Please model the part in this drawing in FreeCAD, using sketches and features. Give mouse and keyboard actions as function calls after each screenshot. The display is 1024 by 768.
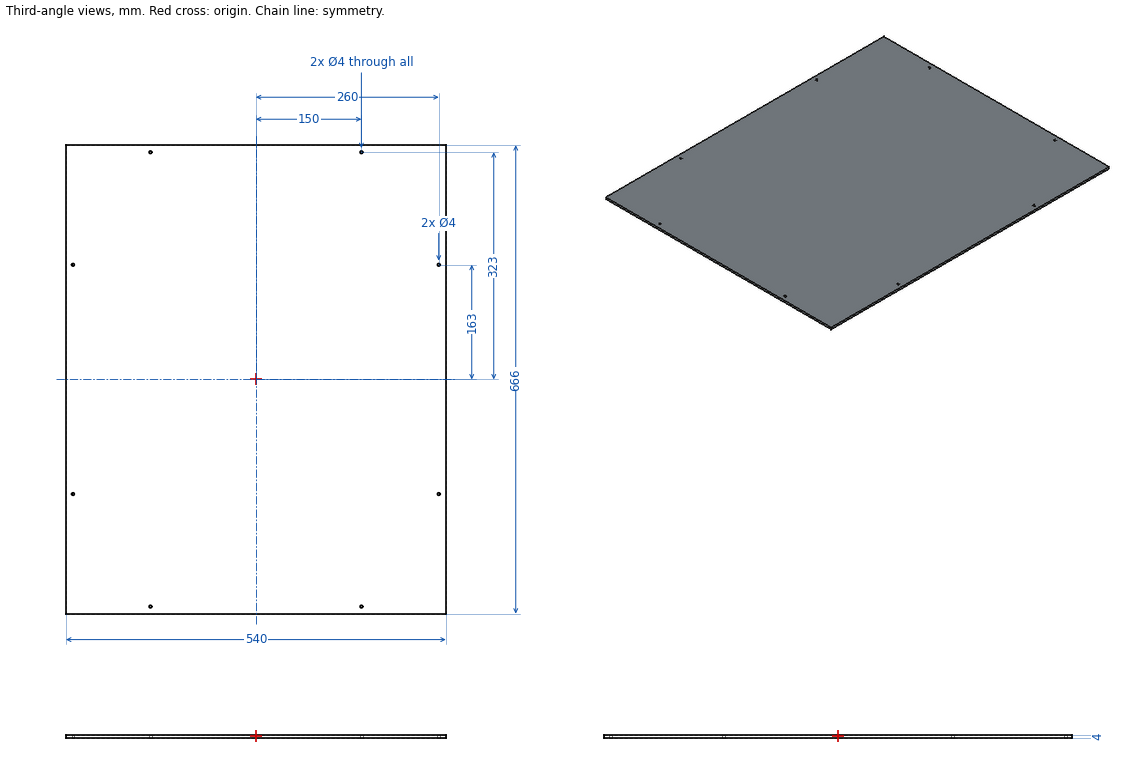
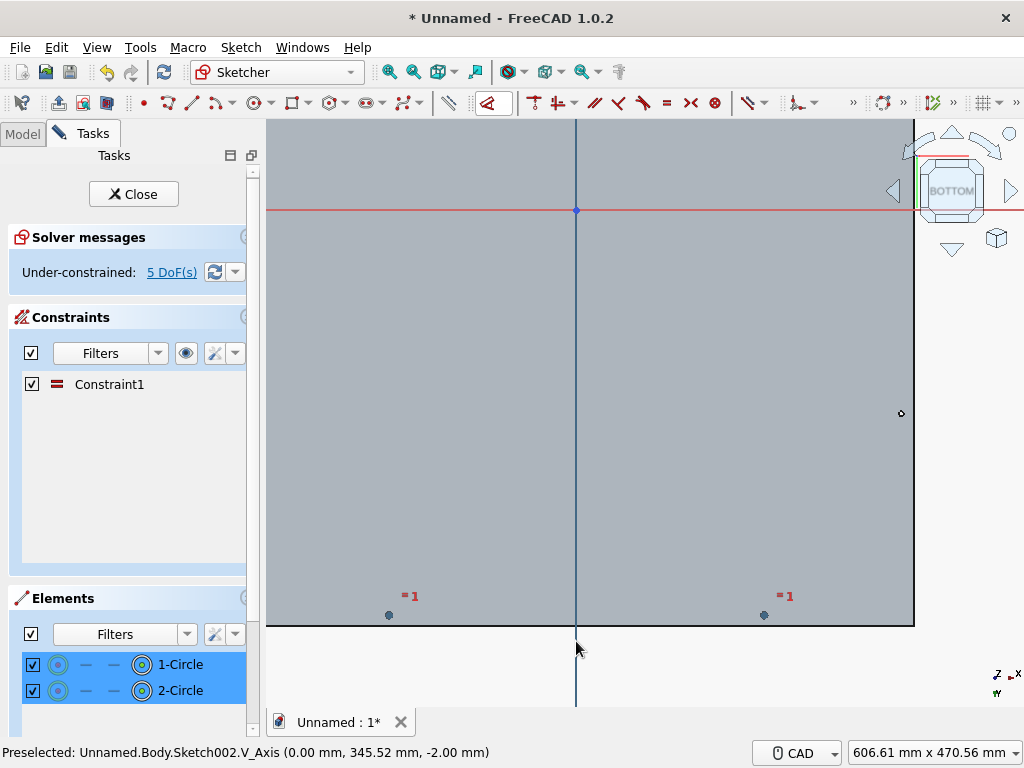
key(s)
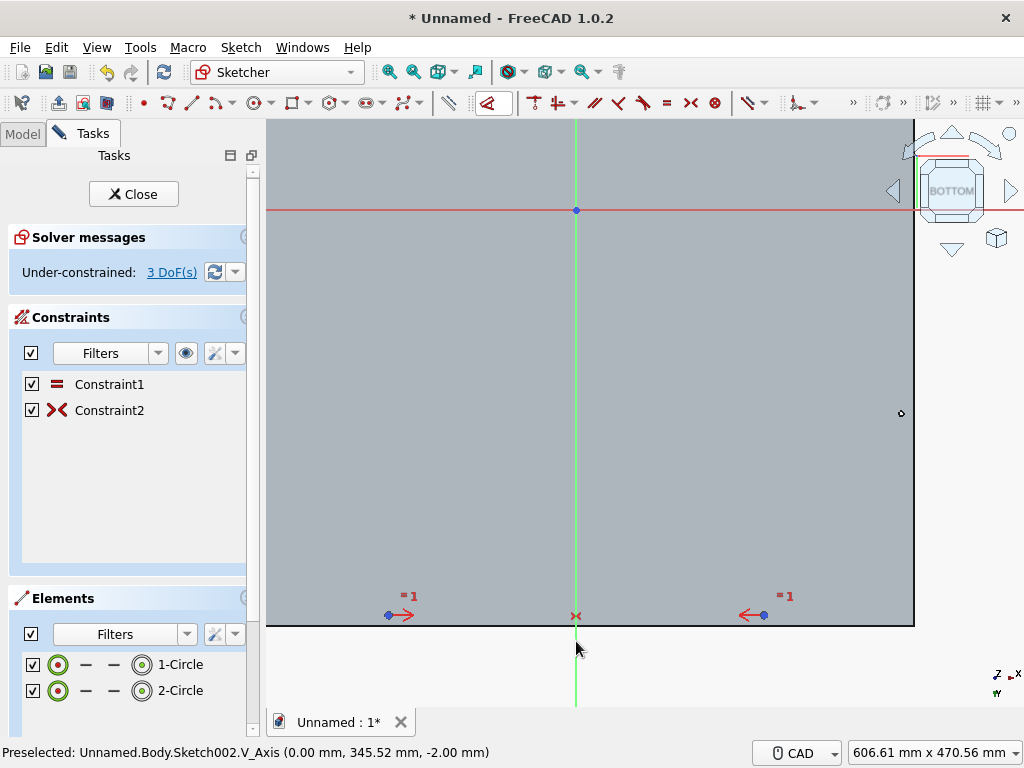
scroll(766, 613, up, 11)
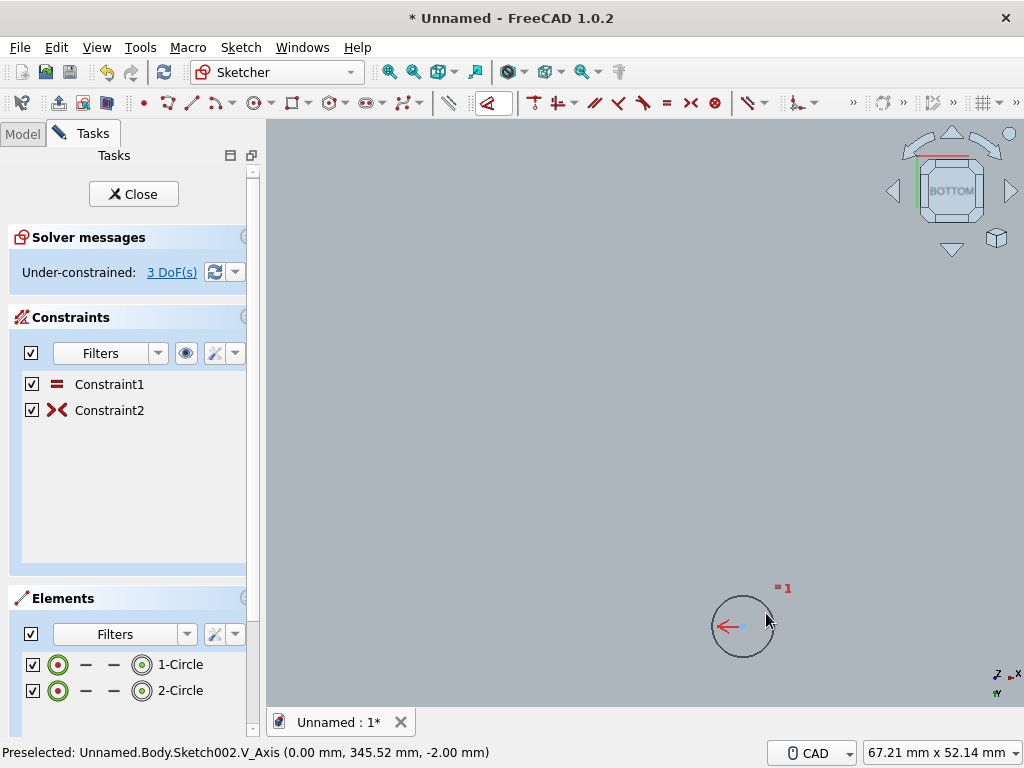
click(765, 605)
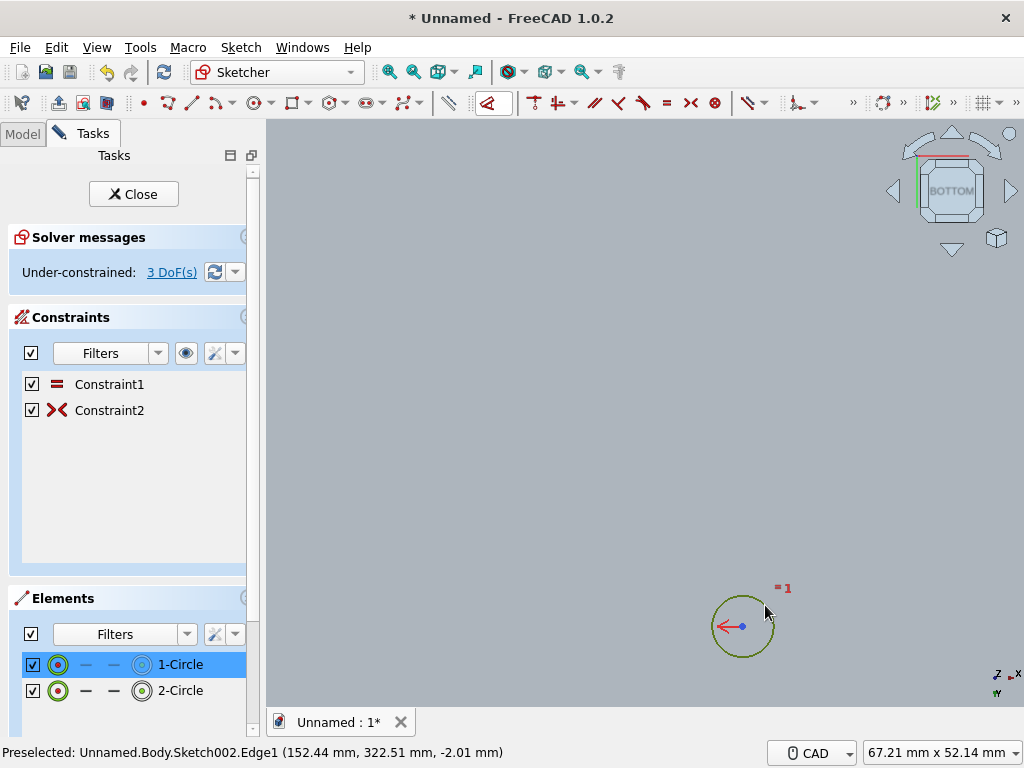
key(k)
key(o)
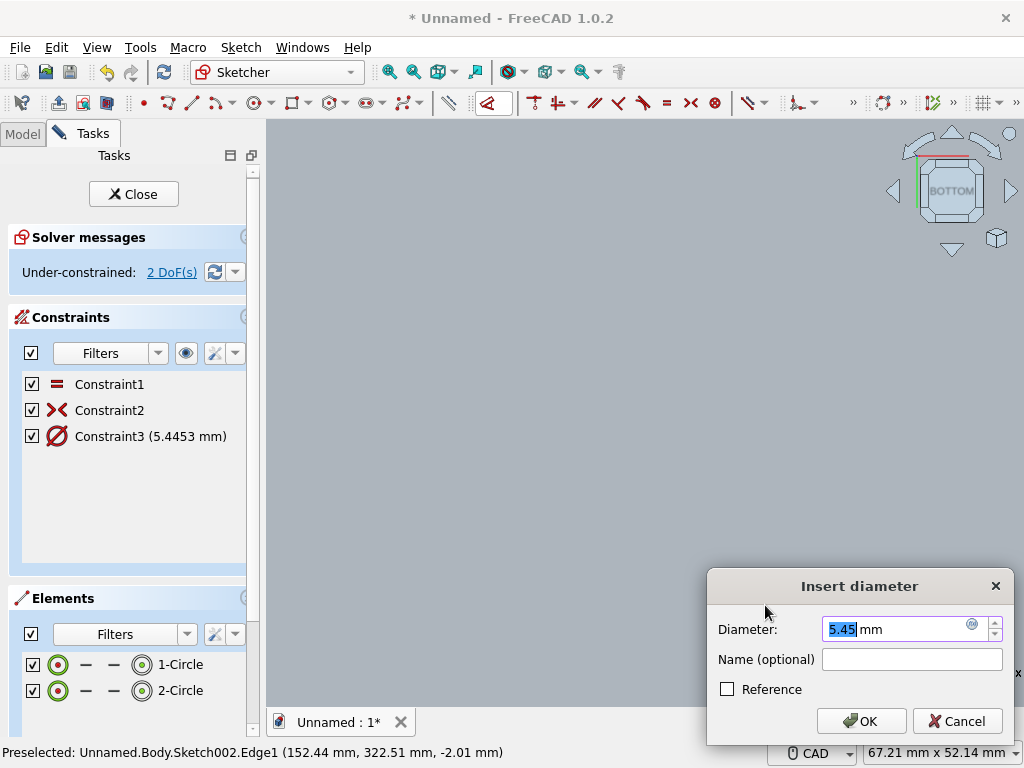
text(4)
key(Return)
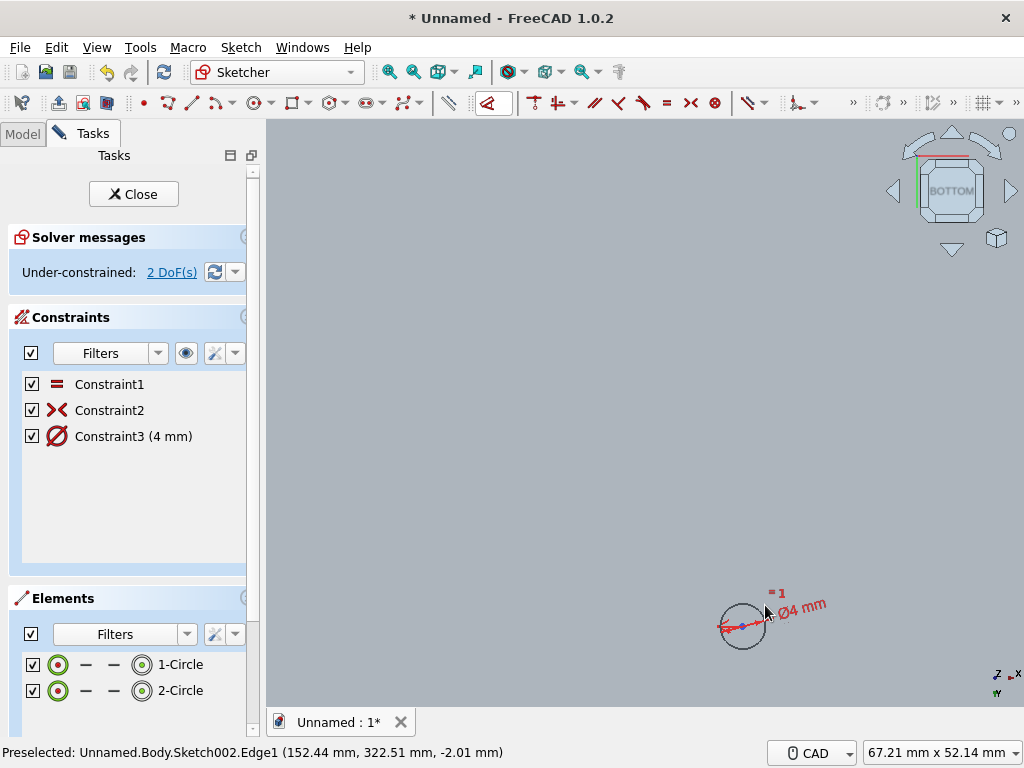
scroll(767, 614, down, 11)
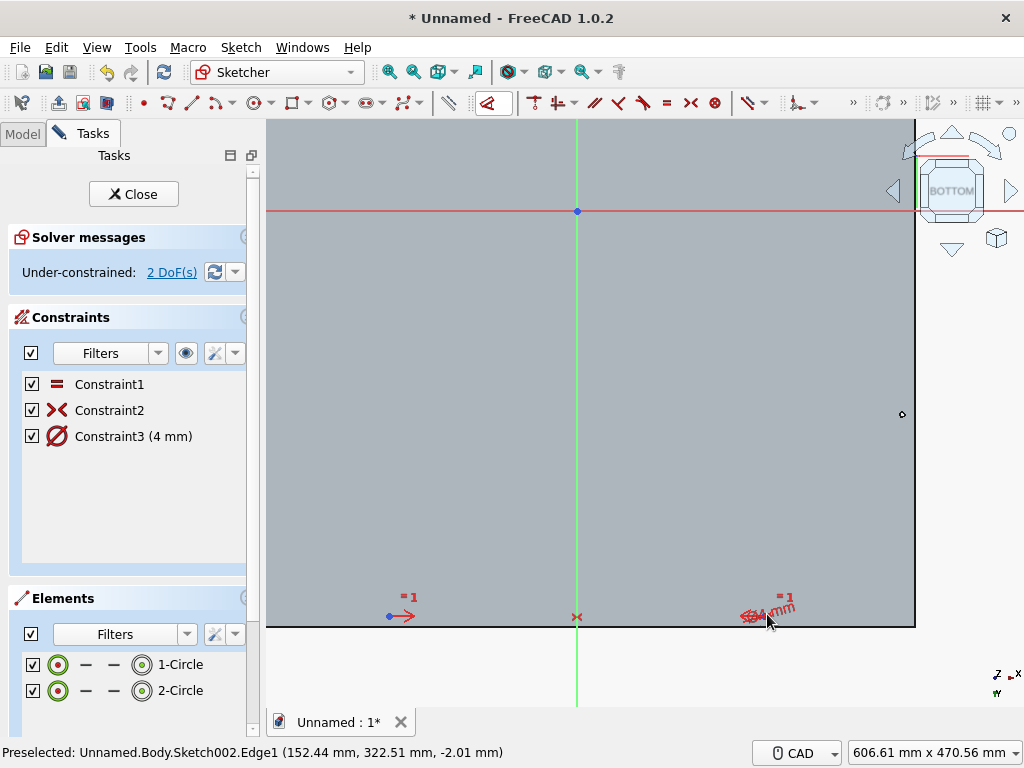
click(765, 616)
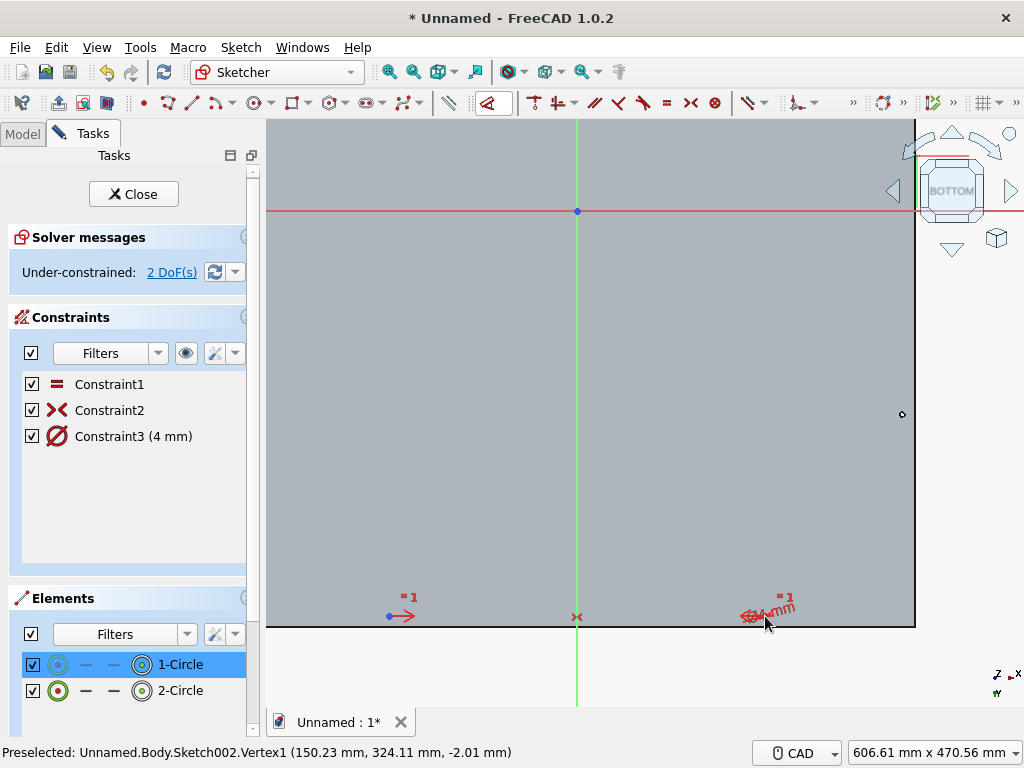
key(l)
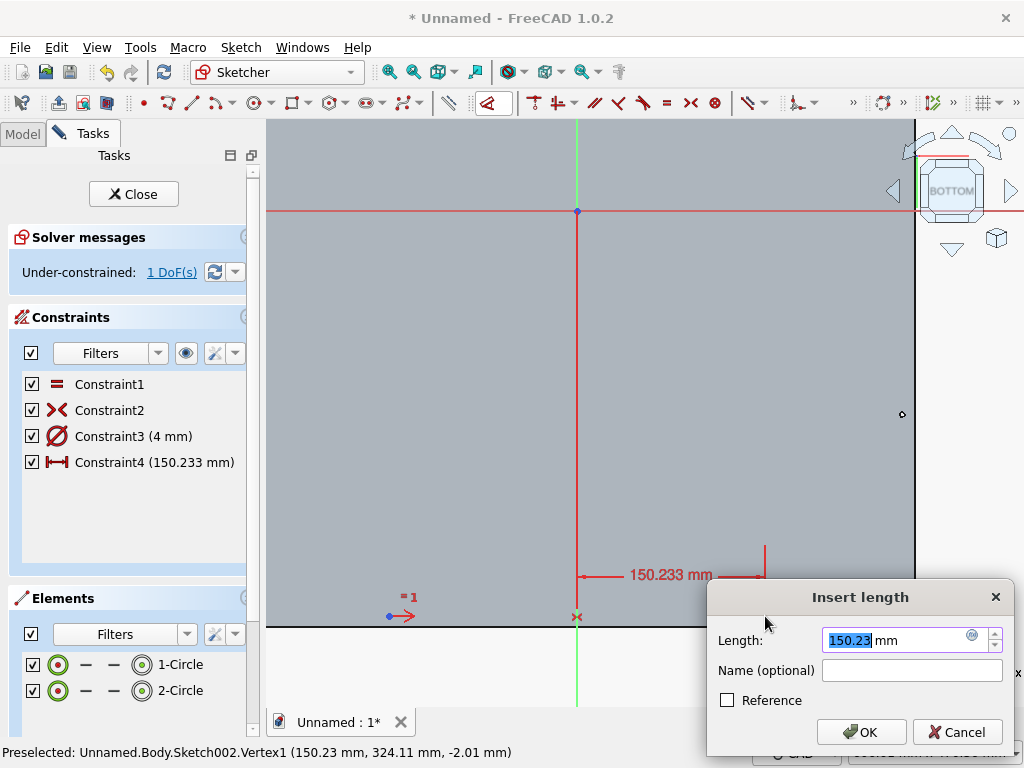
text(150)
key(Return)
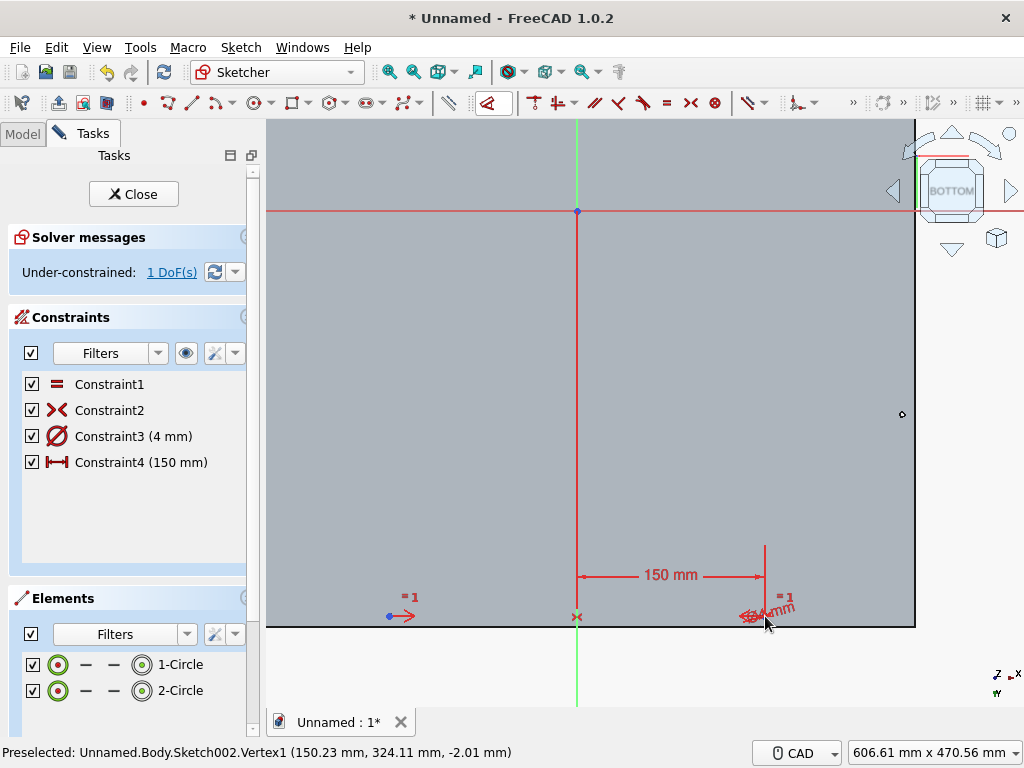
click(765, 616)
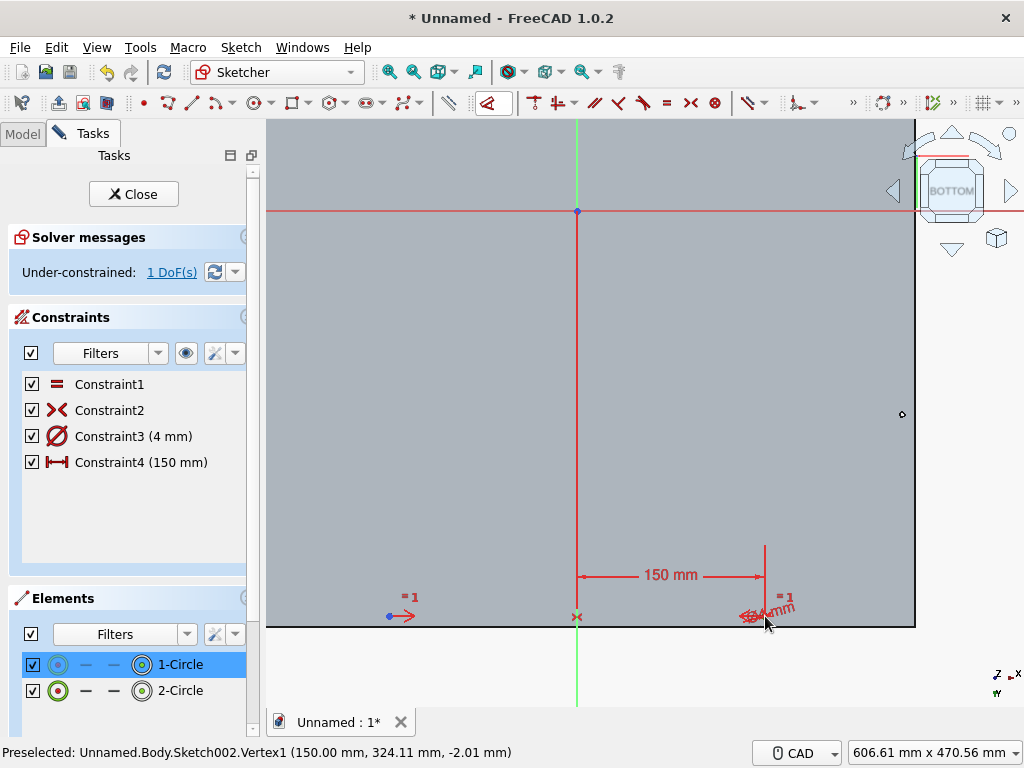
key(i)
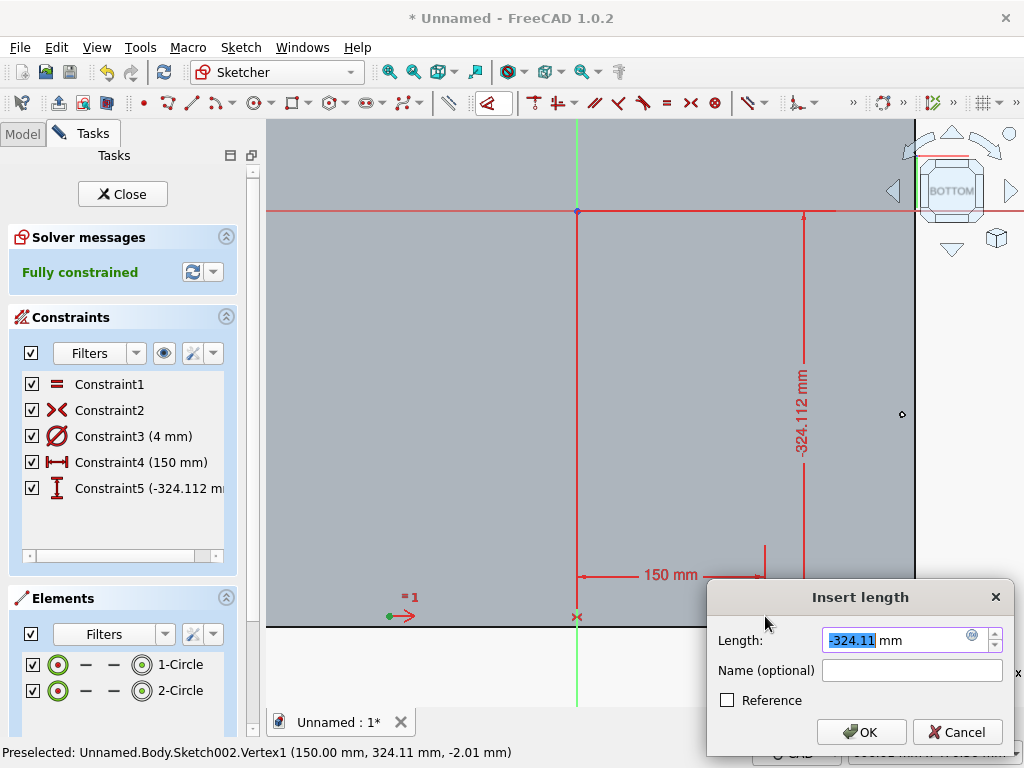
text(-323)
key(Return)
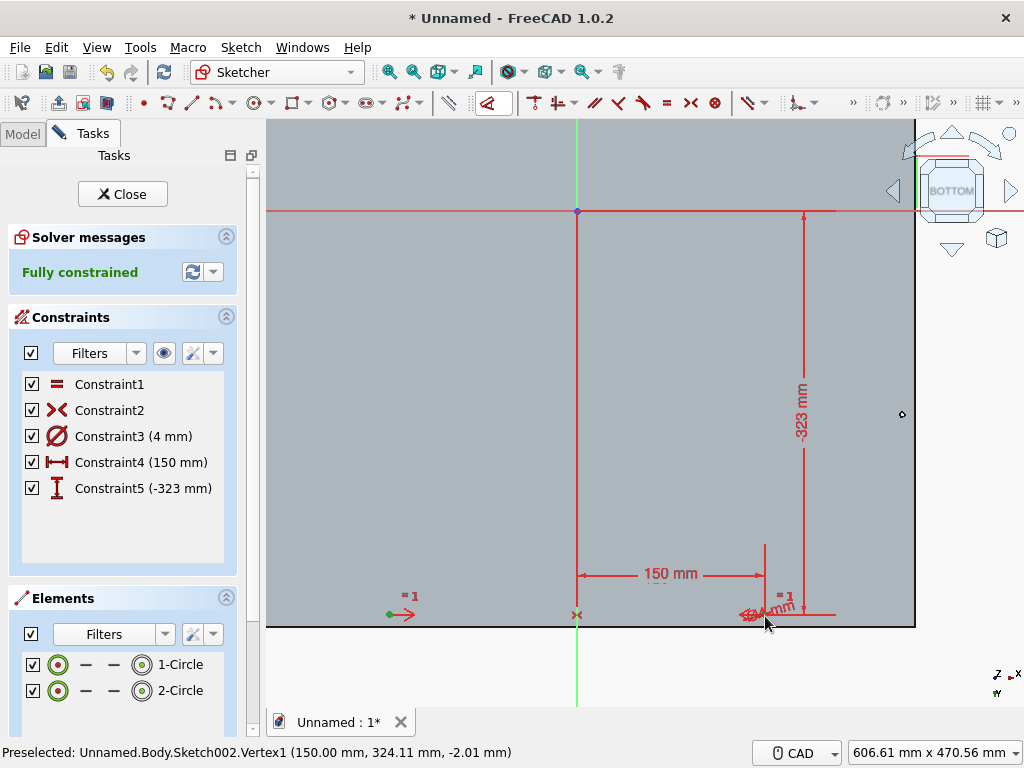
click(123, 194)